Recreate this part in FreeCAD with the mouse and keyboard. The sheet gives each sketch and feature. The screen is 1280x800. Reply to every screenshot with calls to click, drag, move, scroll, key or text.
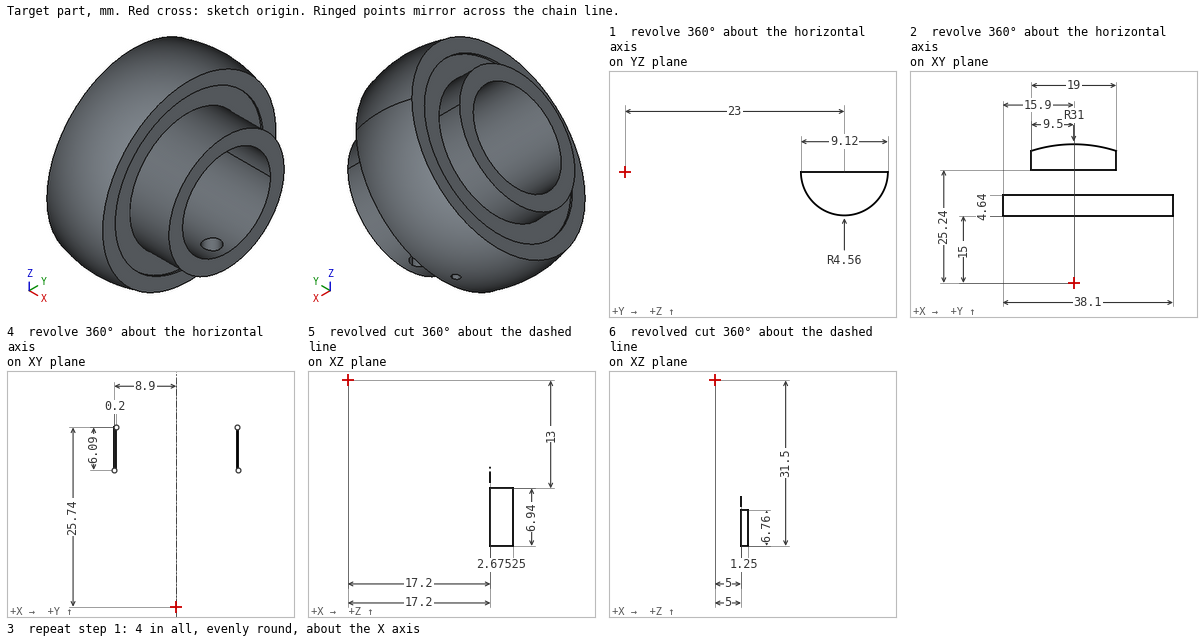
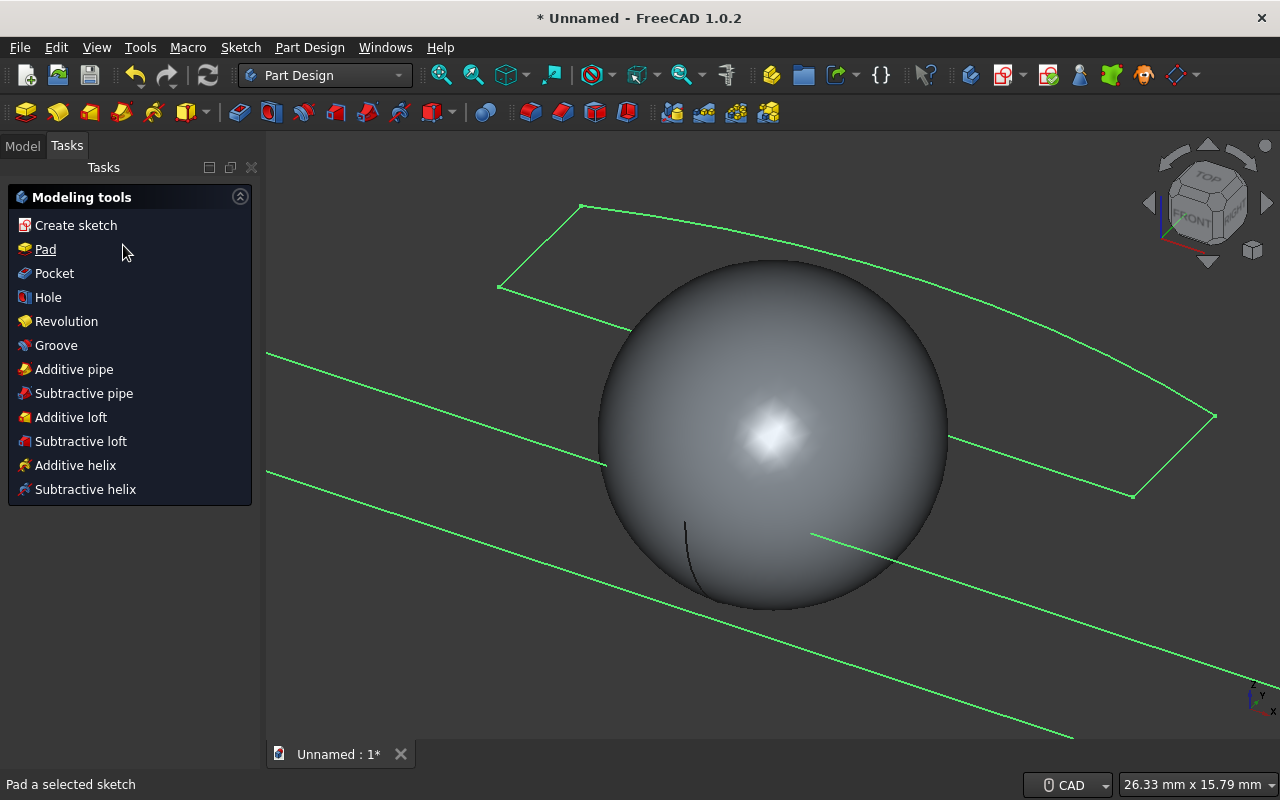
click(58, 112)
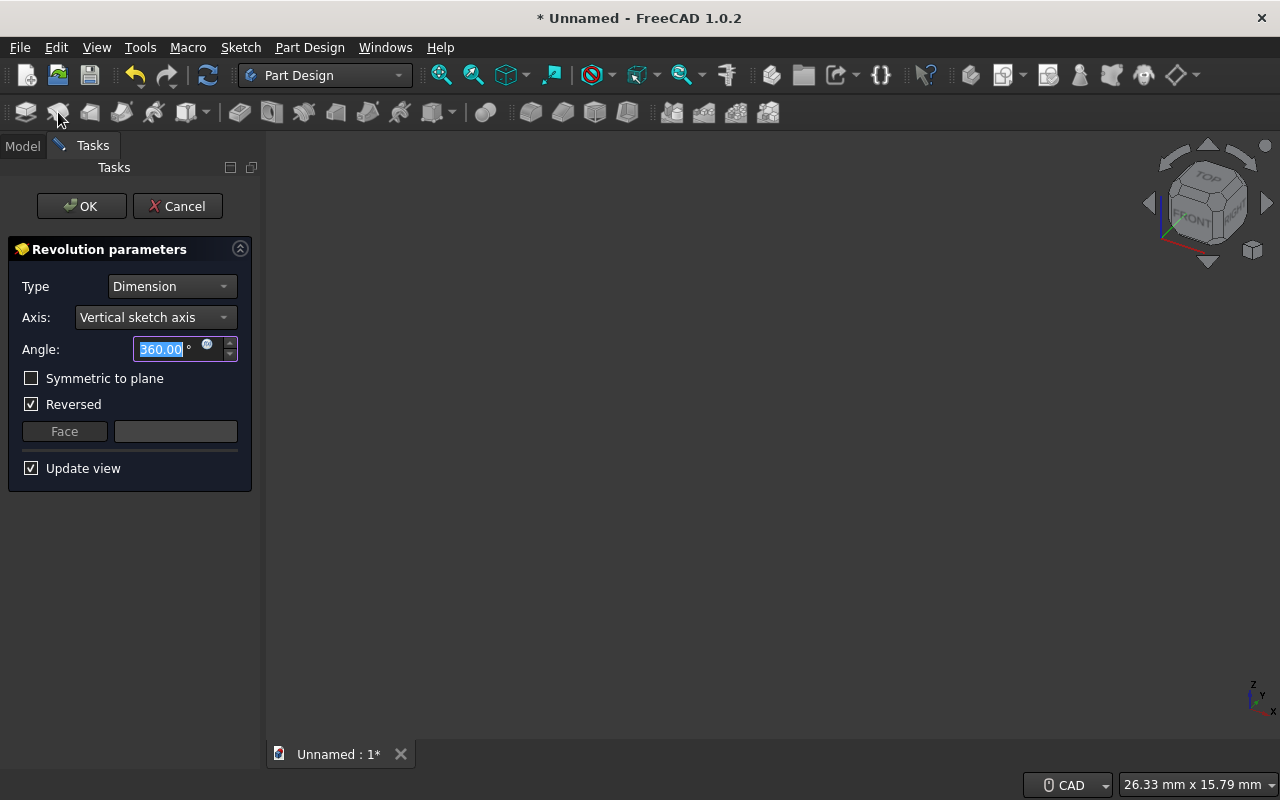
click(156, 318)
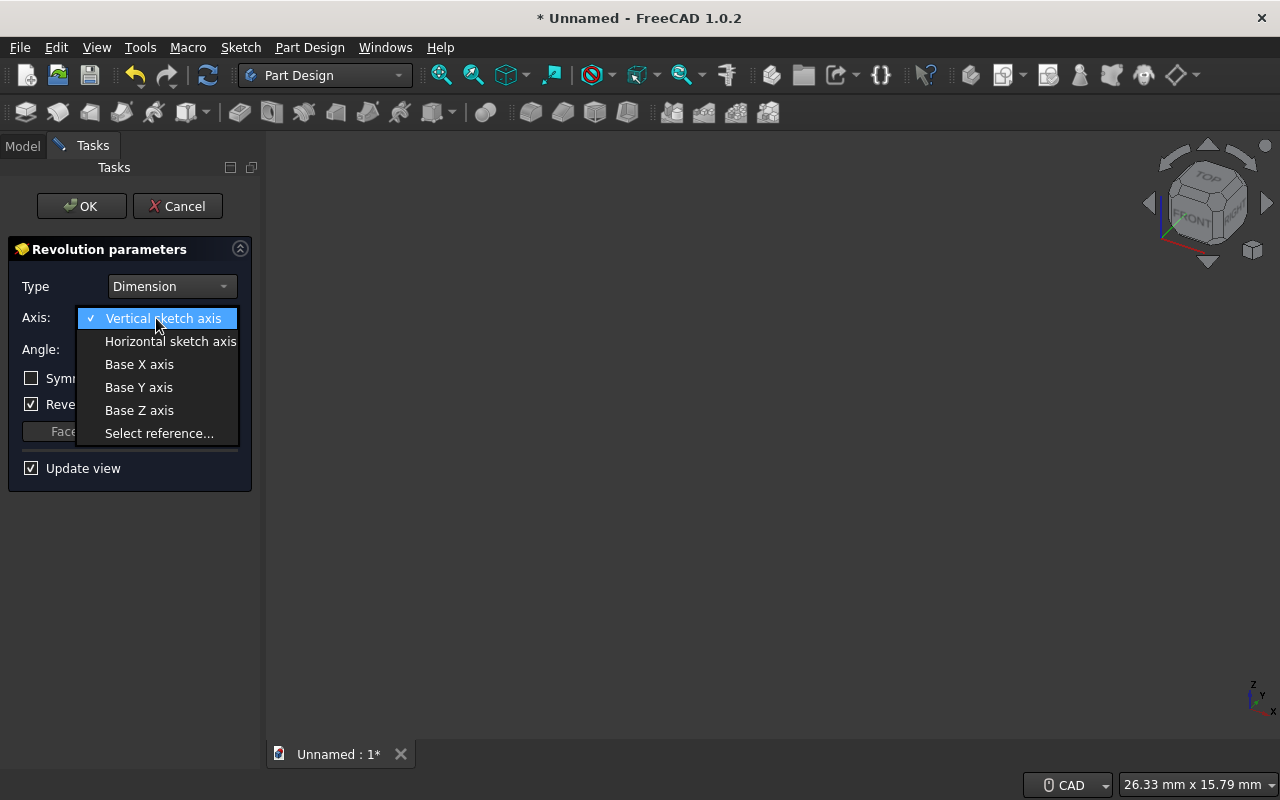
click(156, 342)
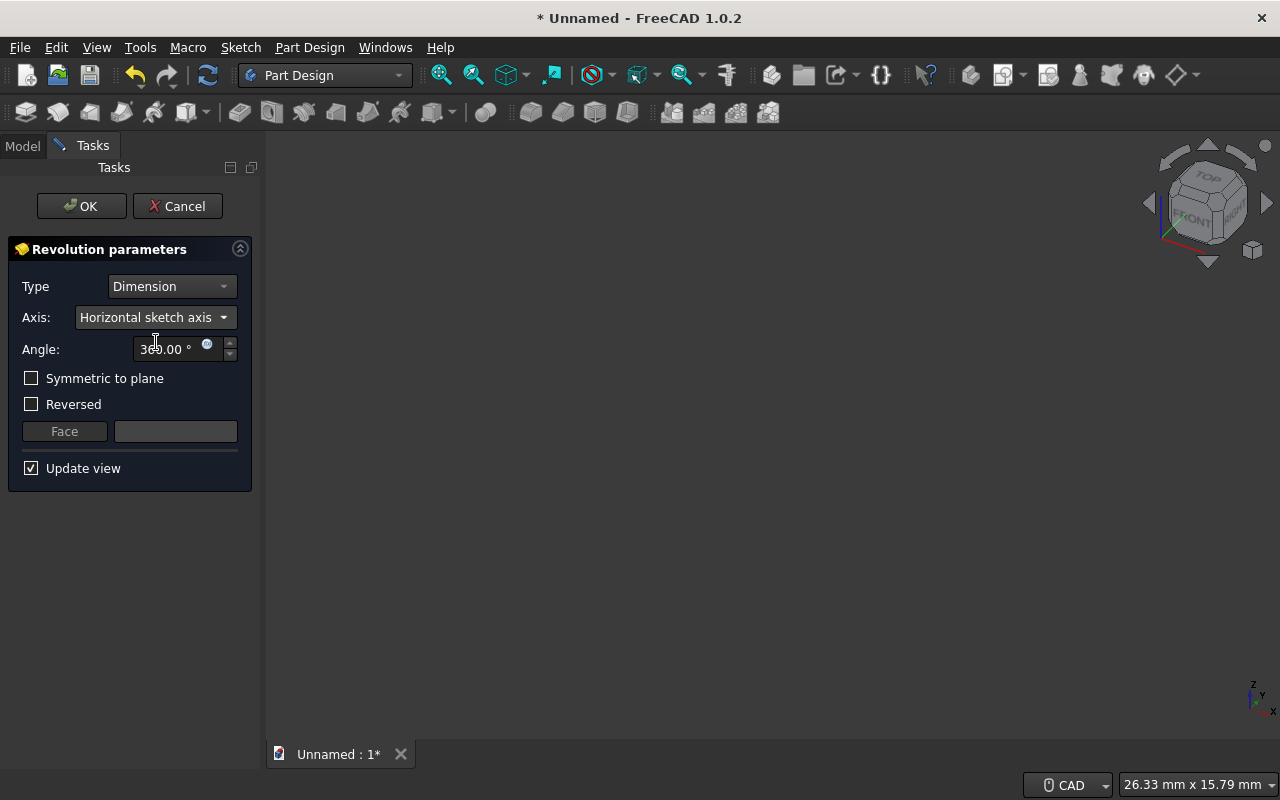
click(82, 206)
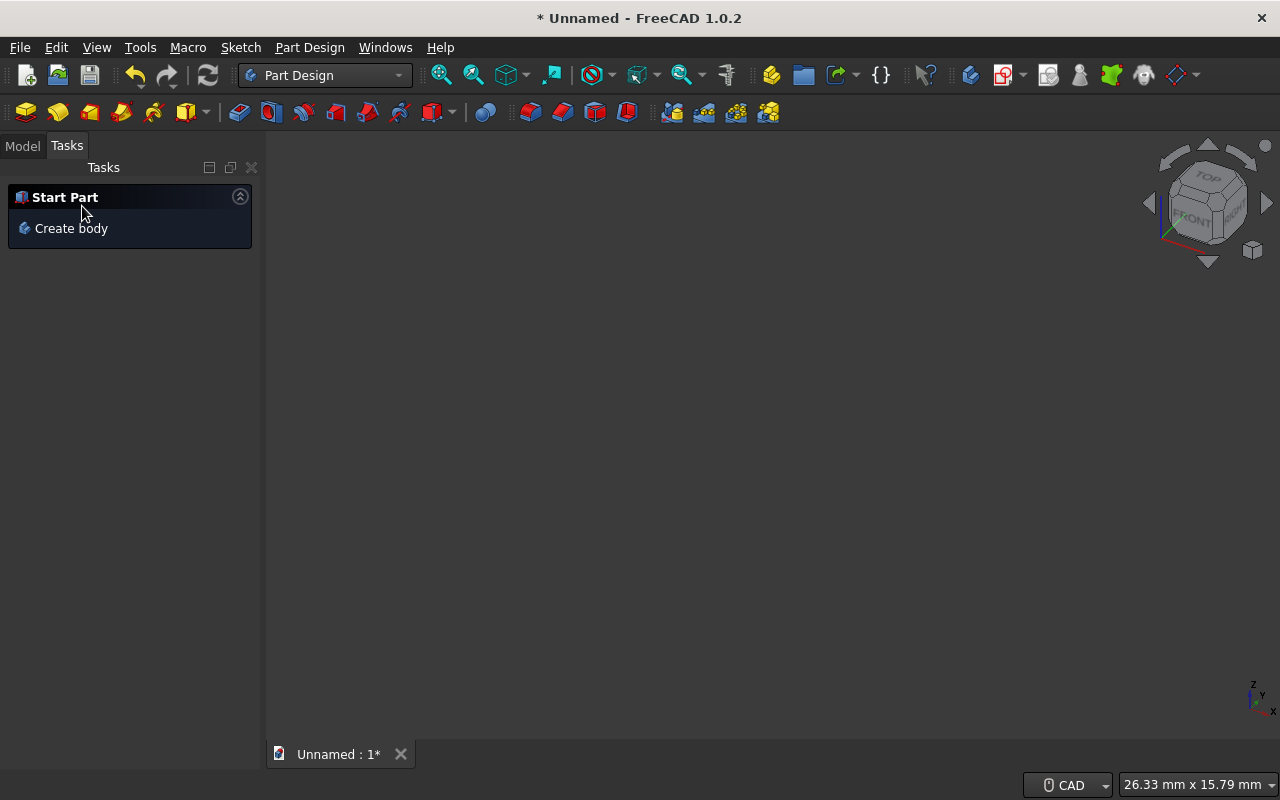
click(442, 76)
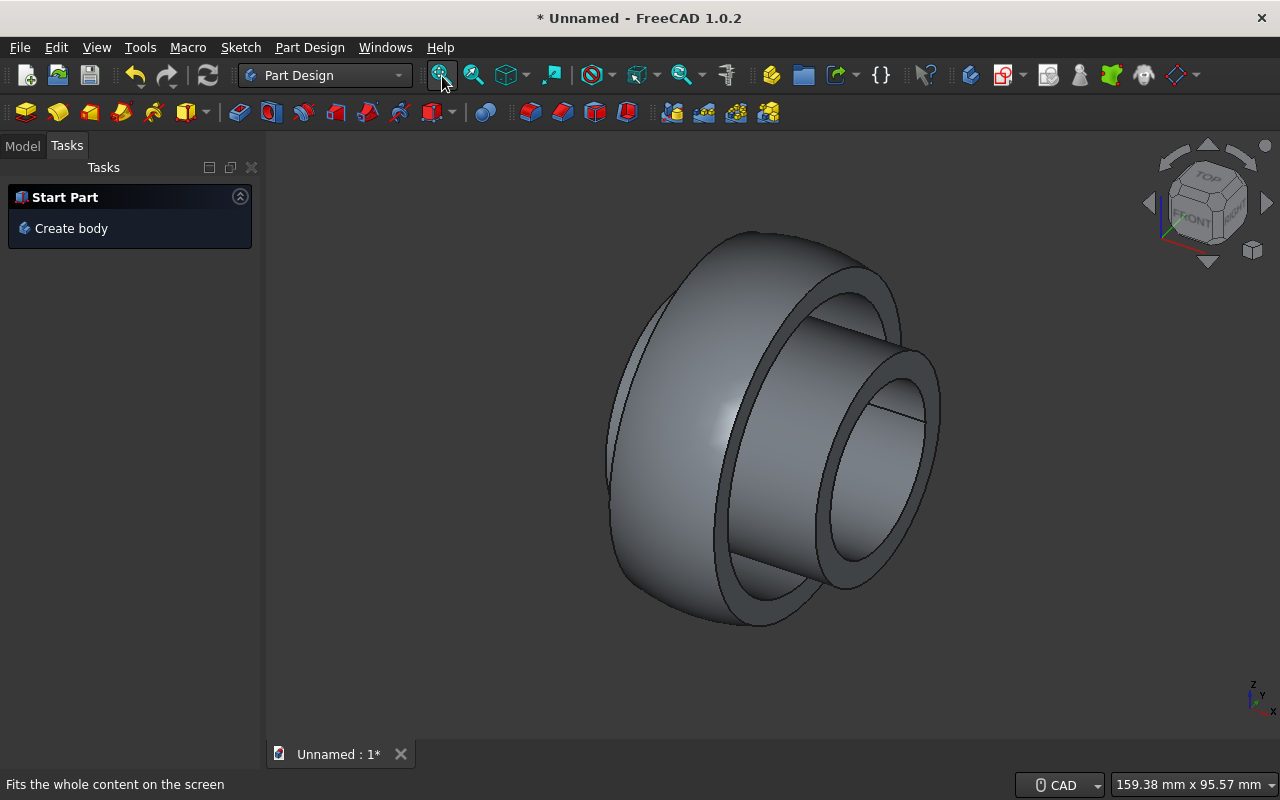
click(23, 145)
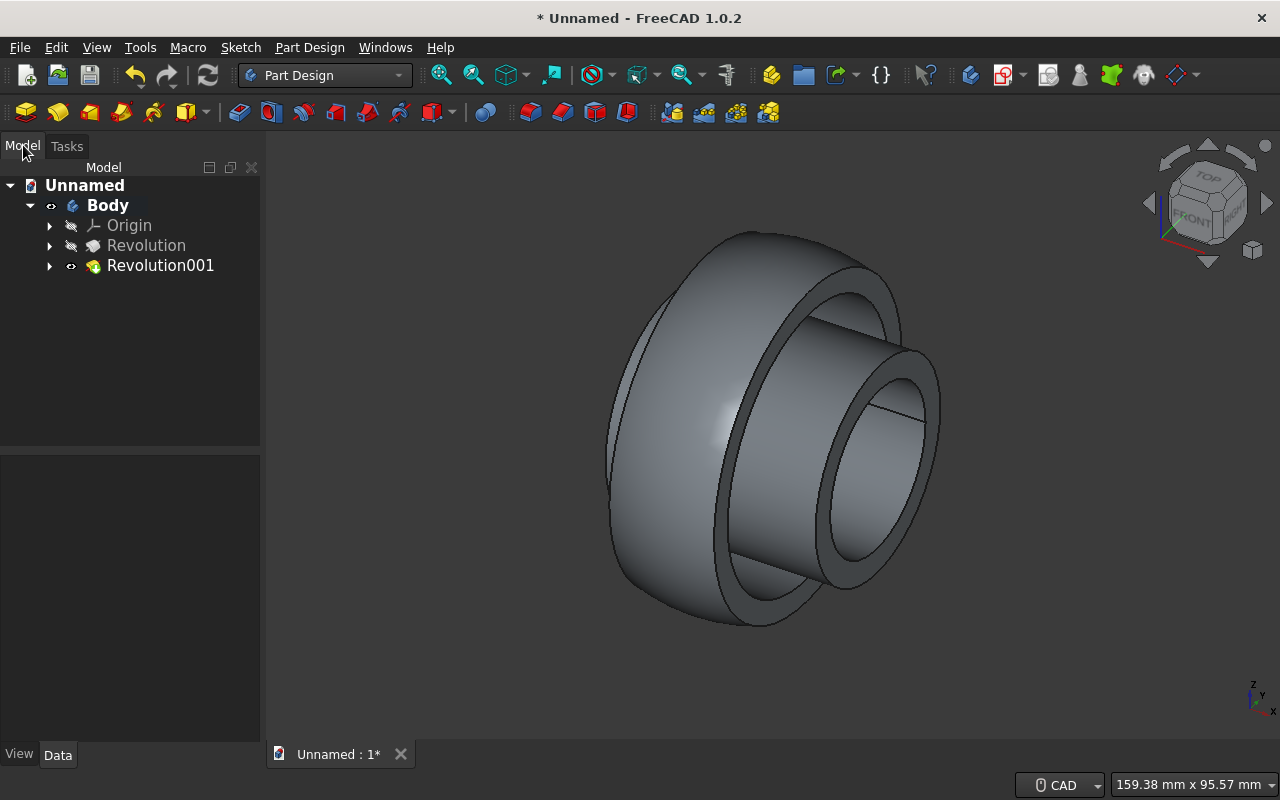
click(116, 246)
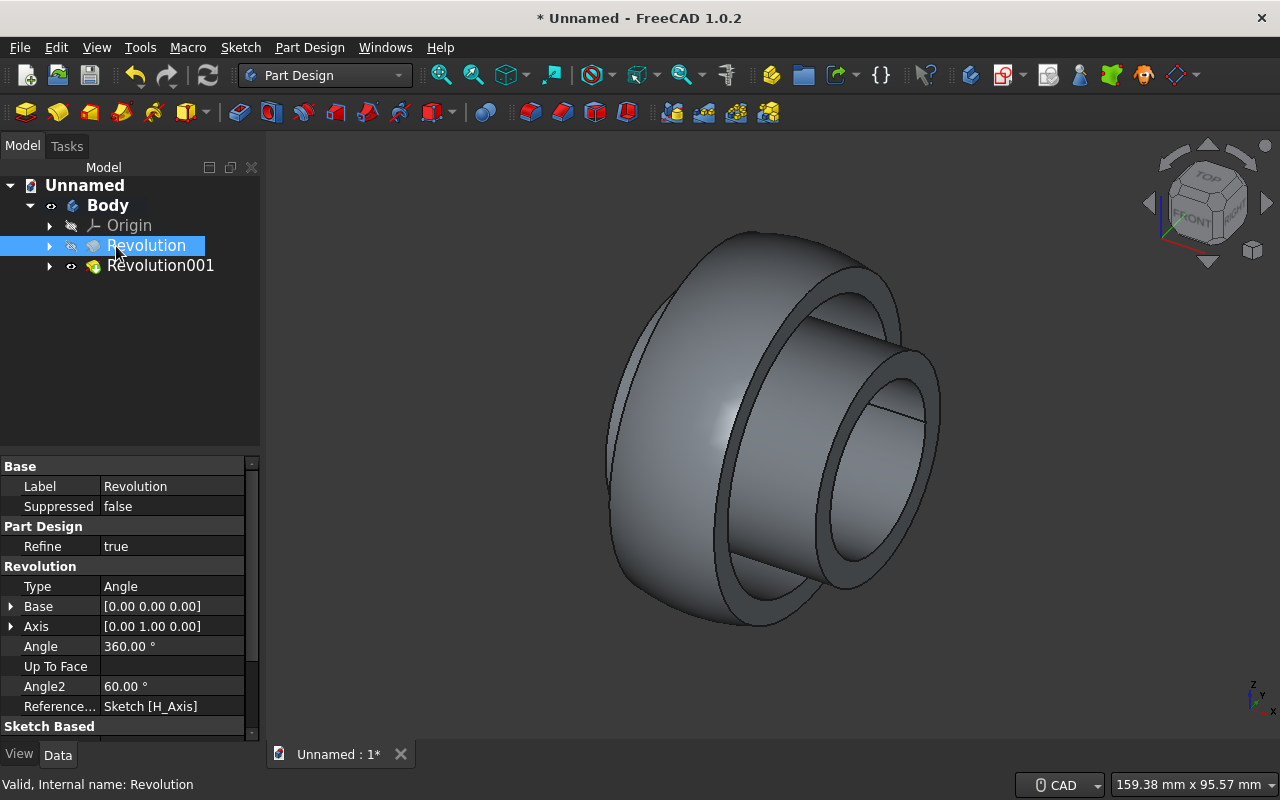
click(736, 112)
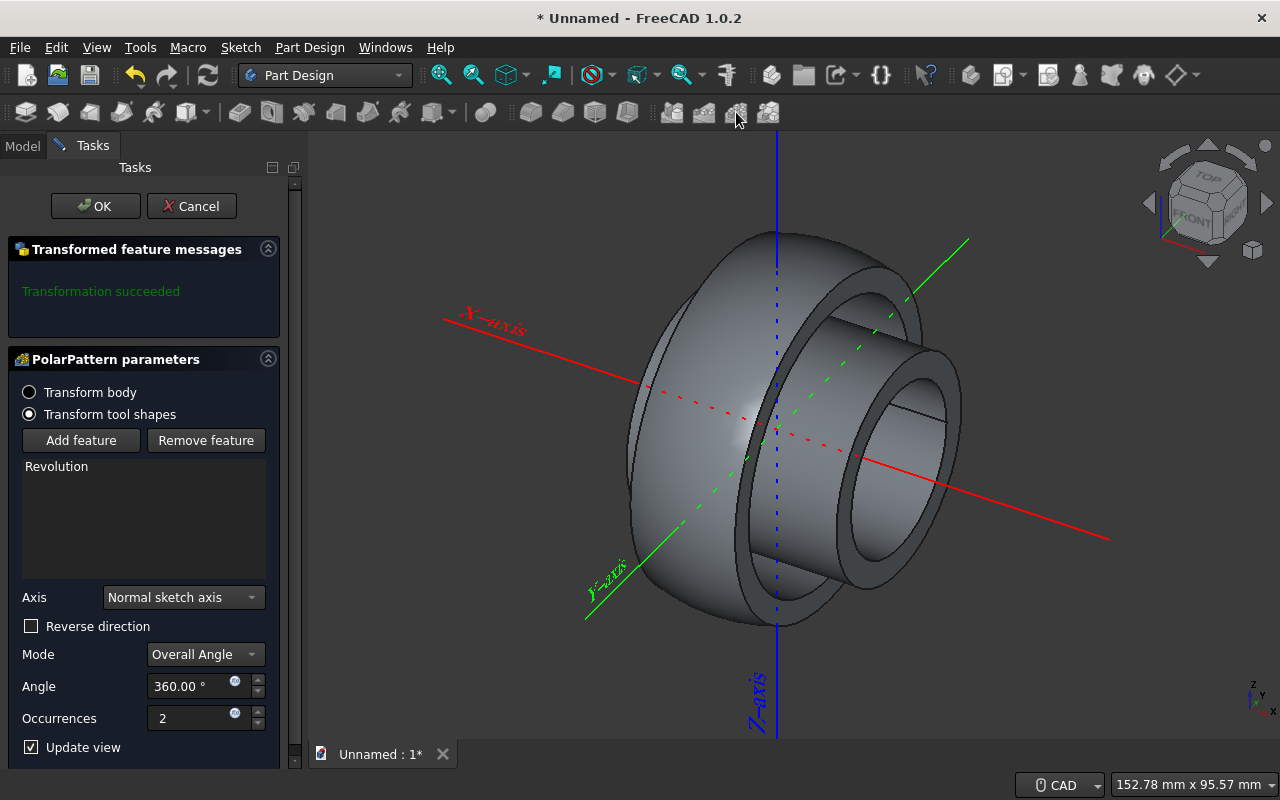
click(184, 598)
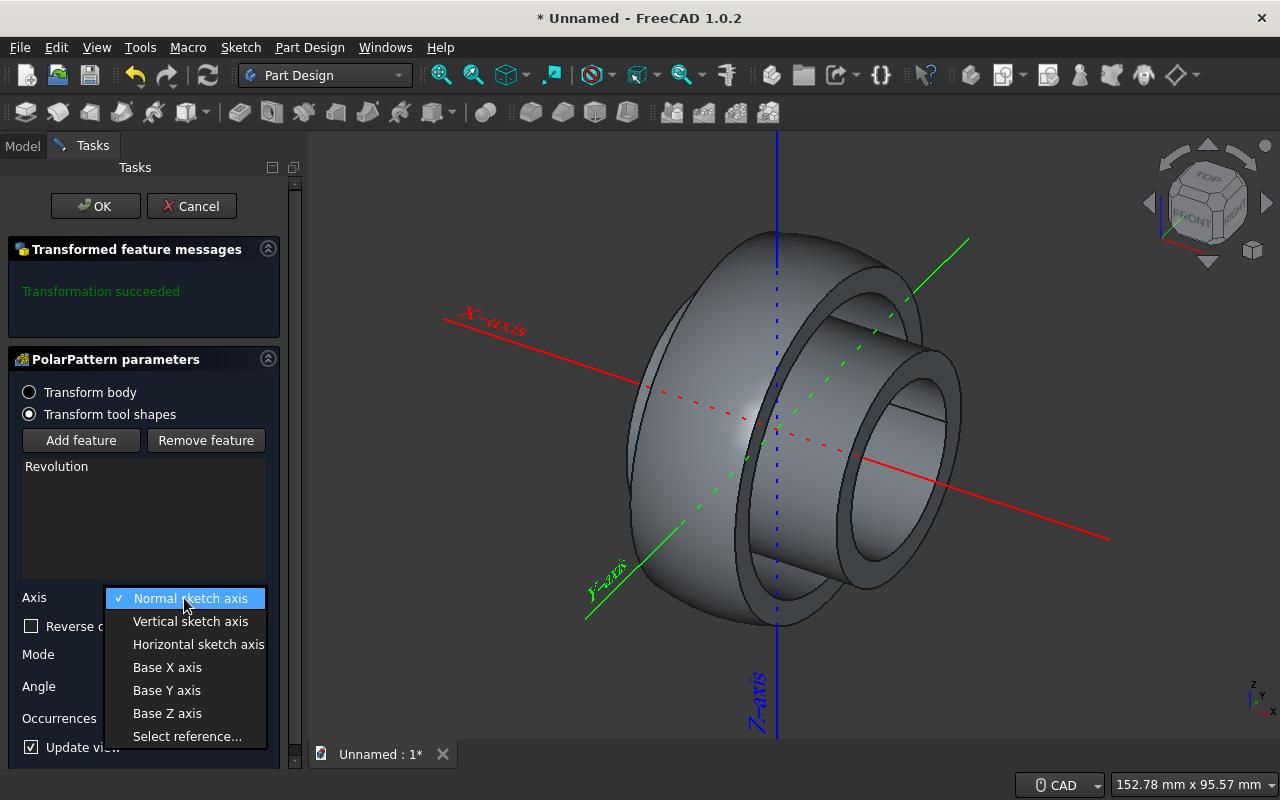
click(184, 668)